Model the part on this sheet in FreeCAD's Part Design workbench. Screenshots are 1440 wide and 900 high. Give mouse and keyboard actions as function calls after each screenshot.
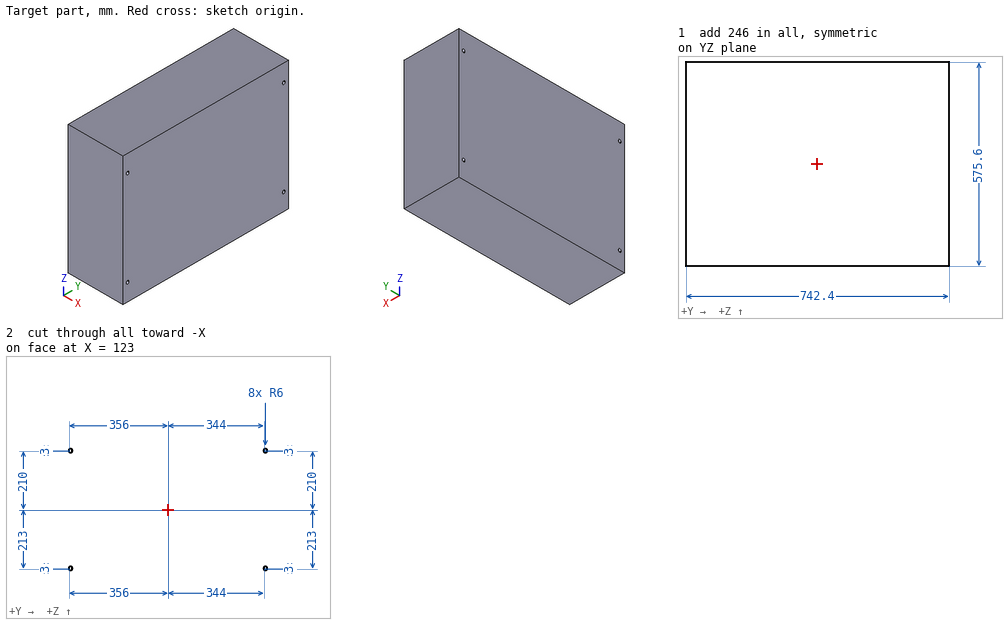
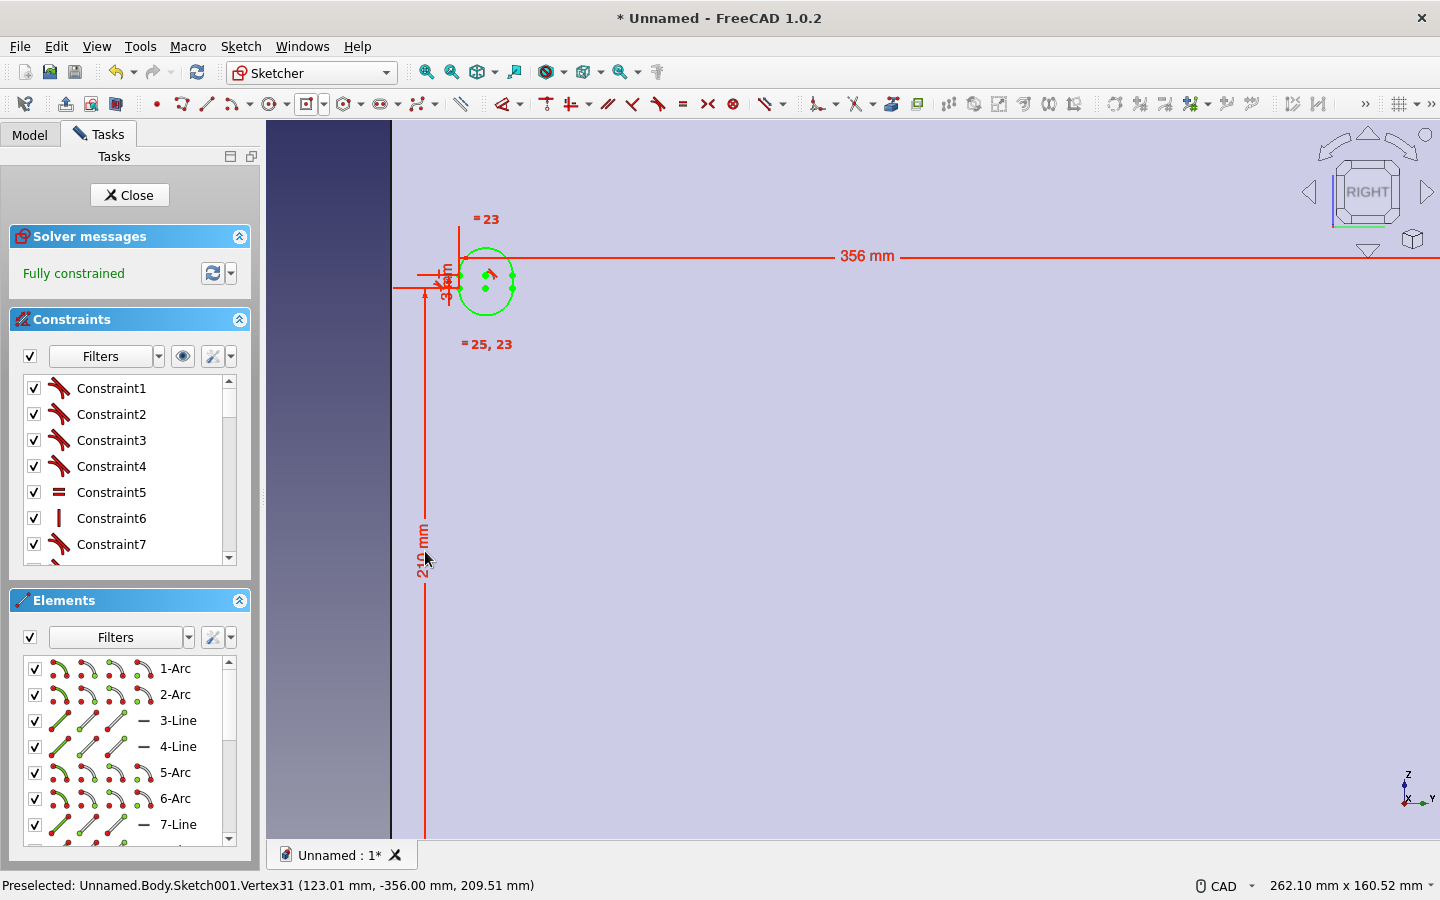
click(130, 195)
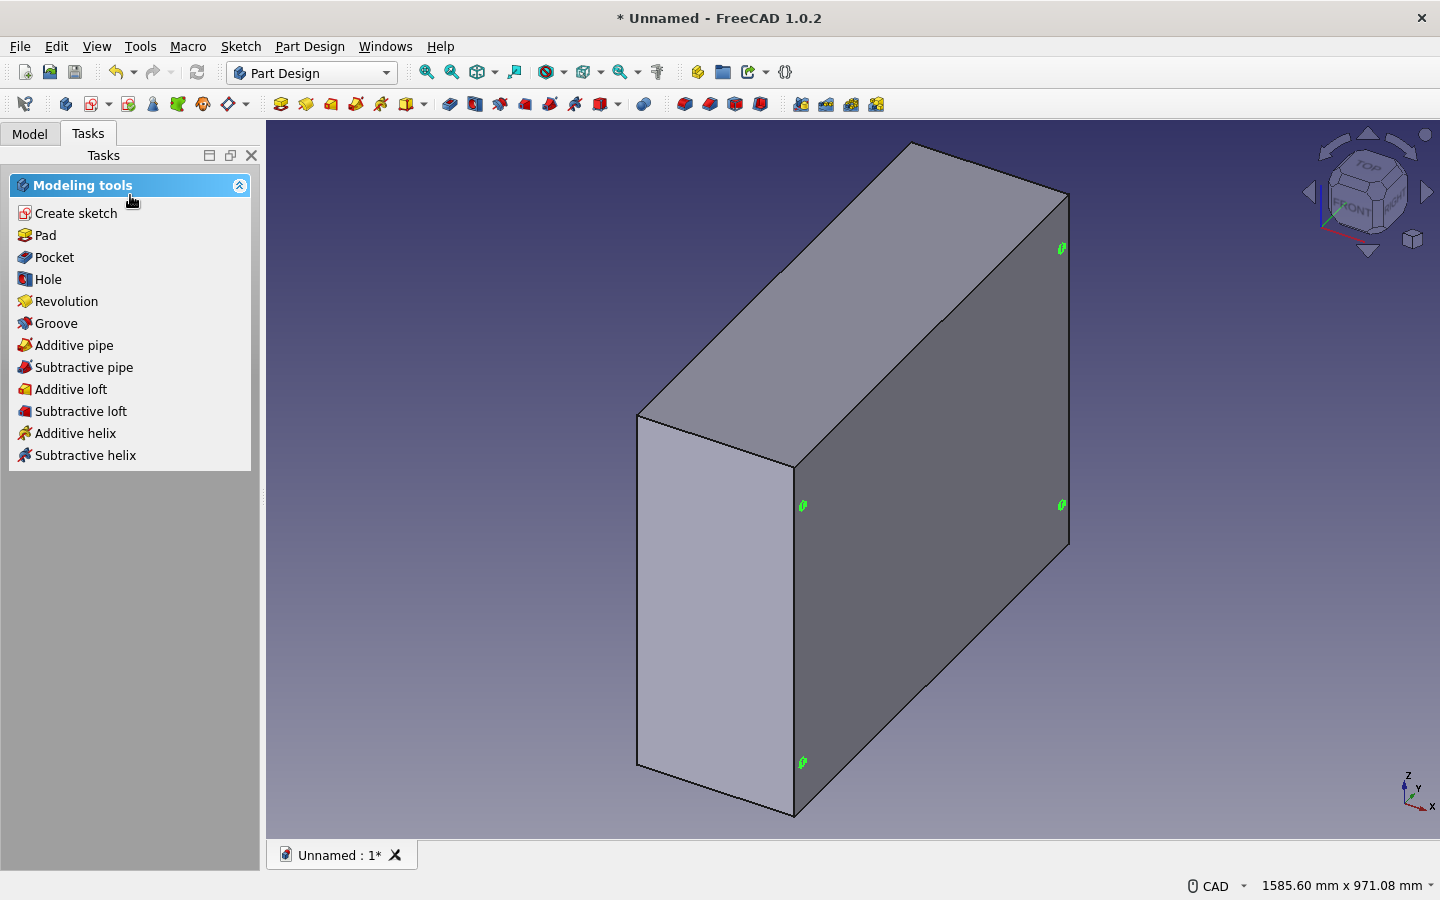
click(450, 104)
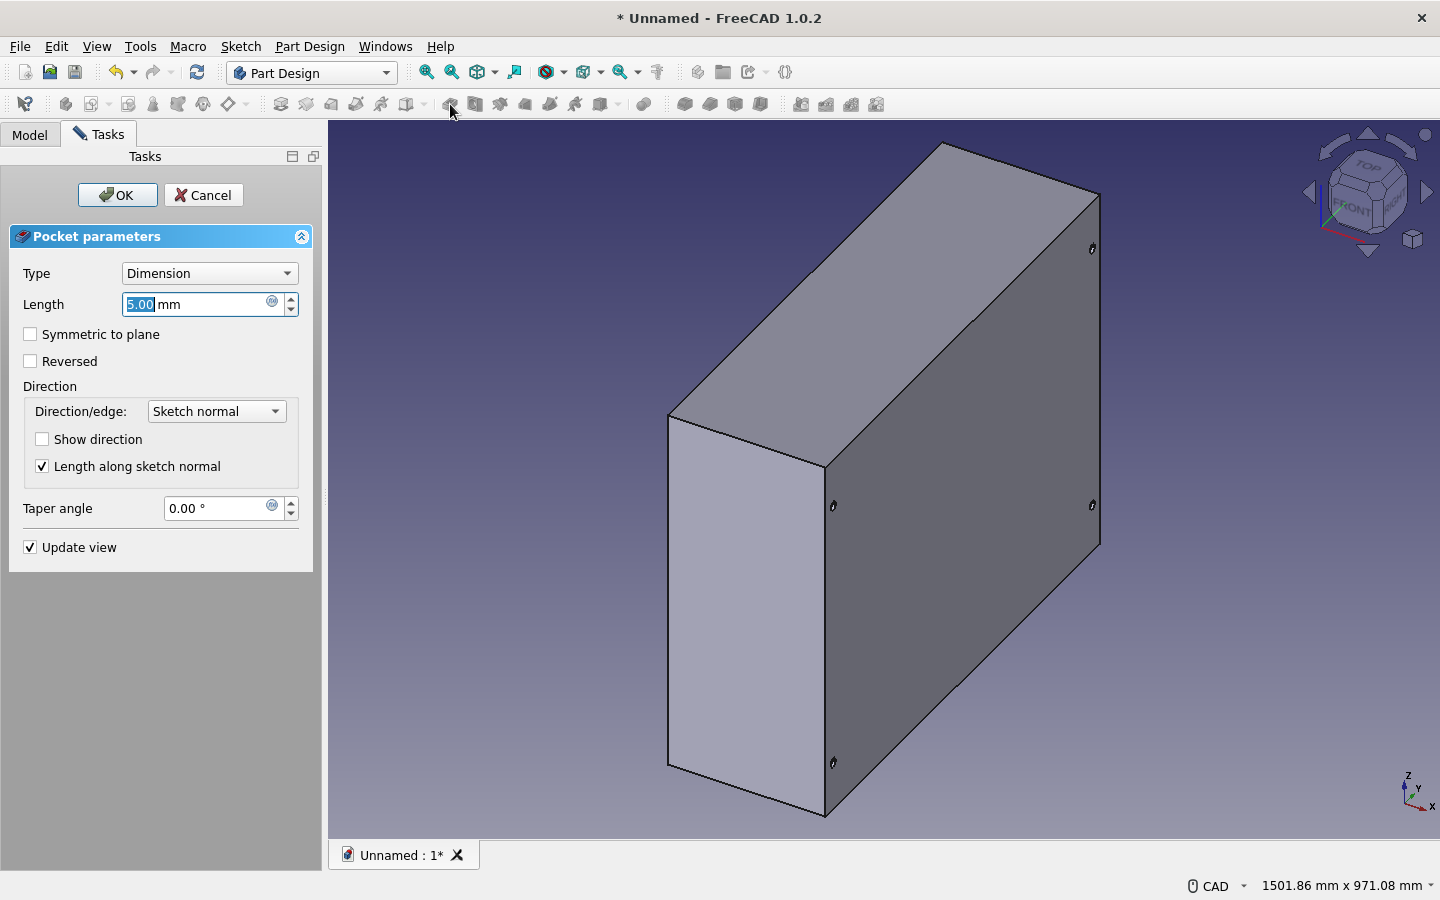
click(210, 274)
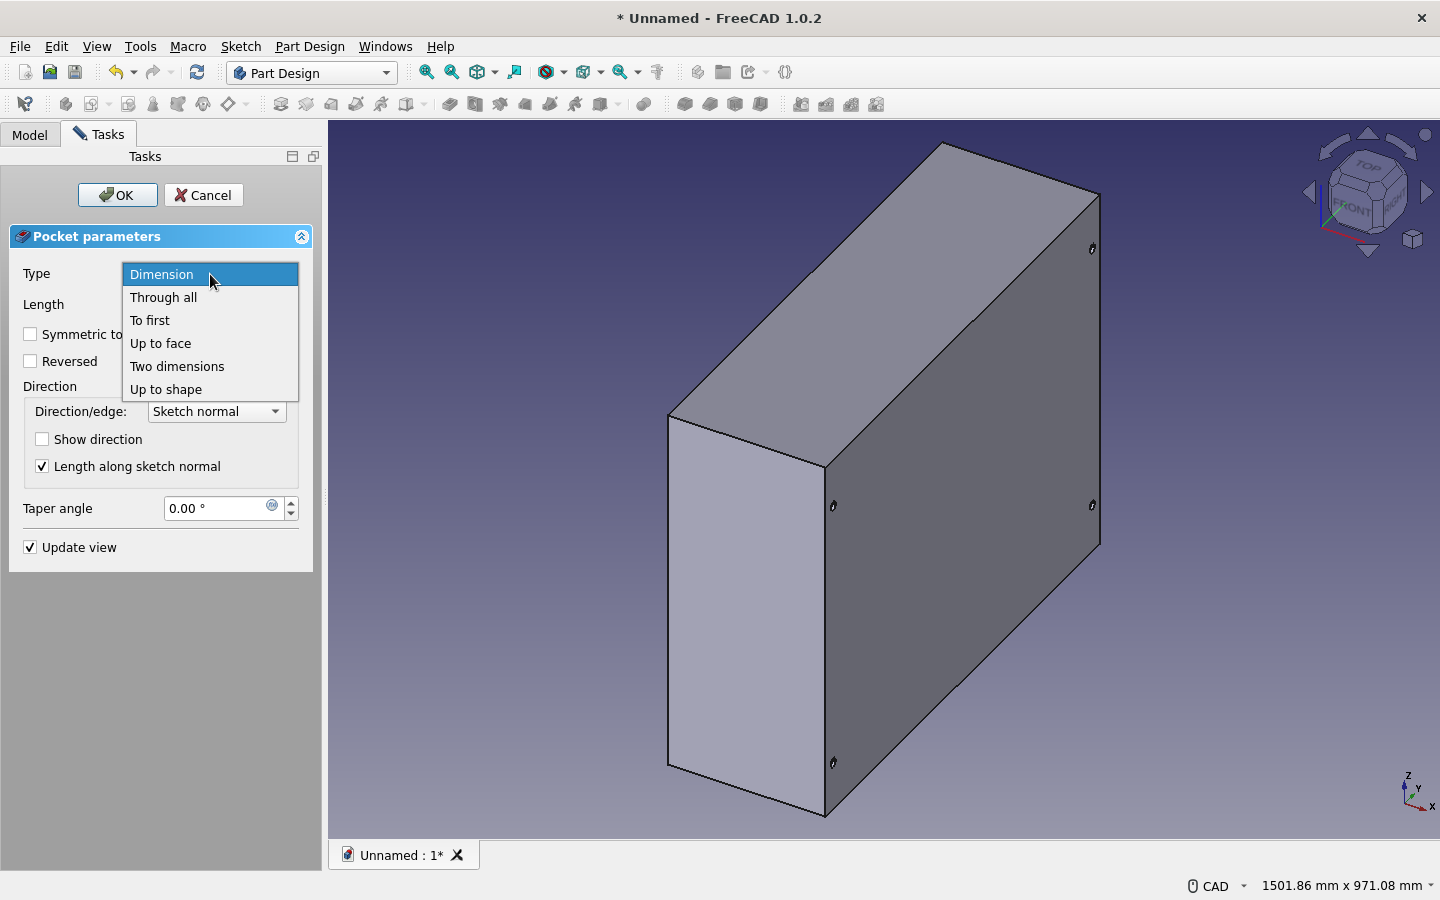
click(208, 298)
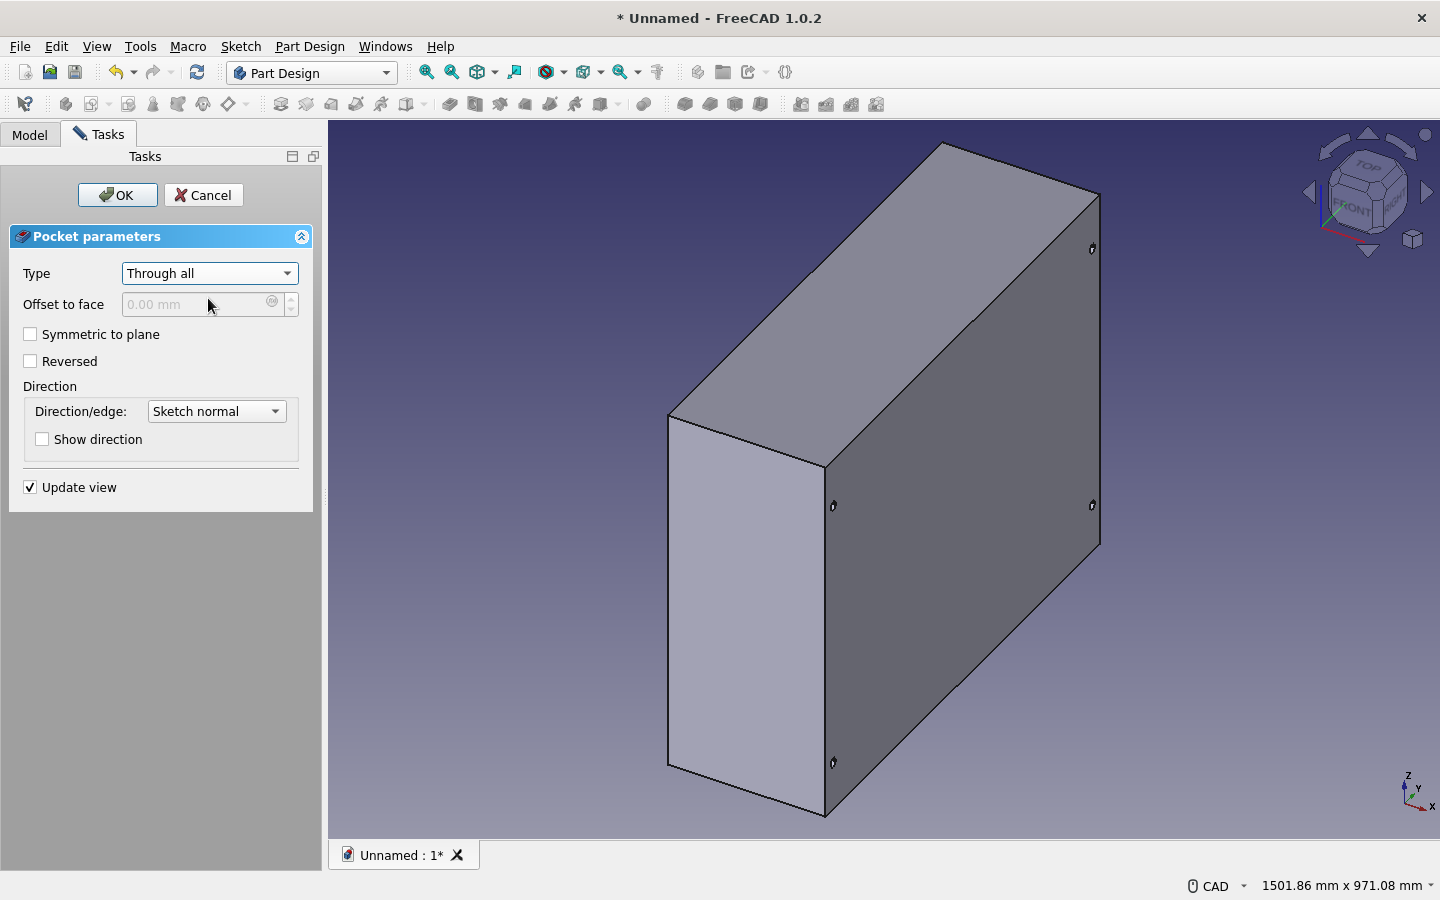
click(118, 195)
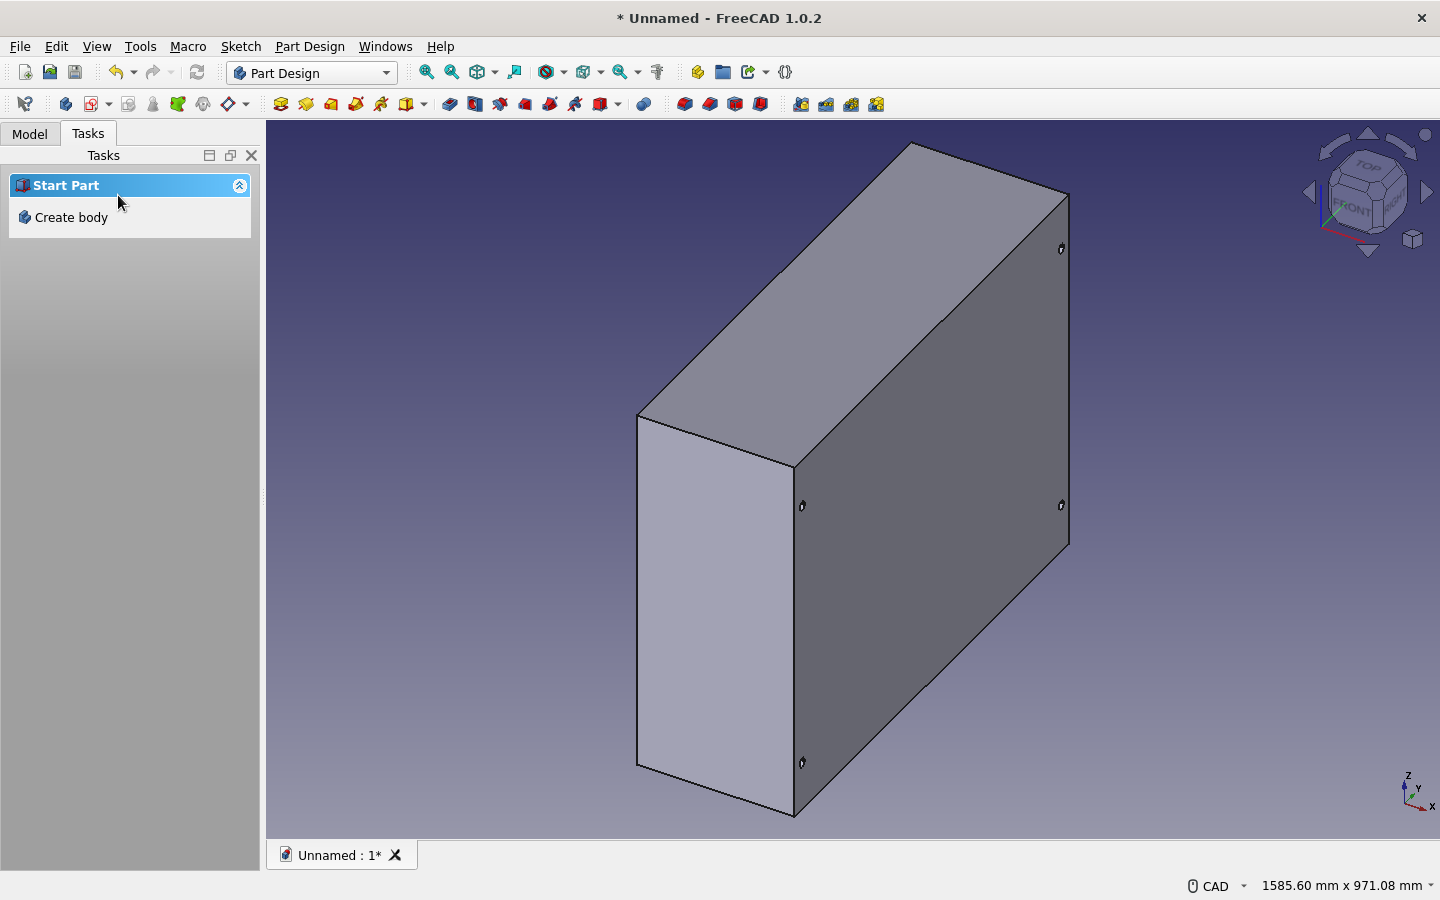
key(0)